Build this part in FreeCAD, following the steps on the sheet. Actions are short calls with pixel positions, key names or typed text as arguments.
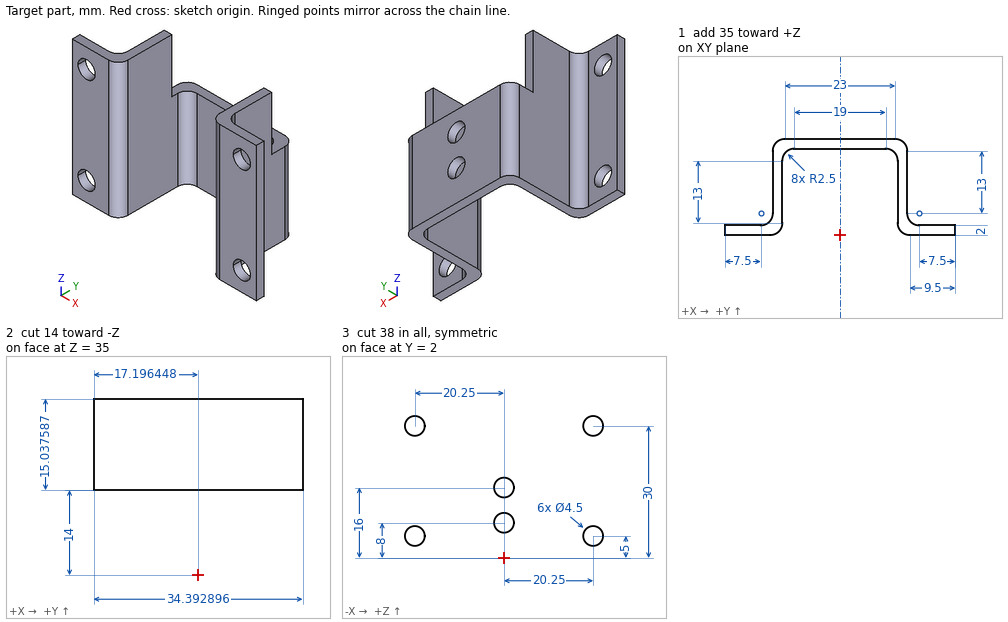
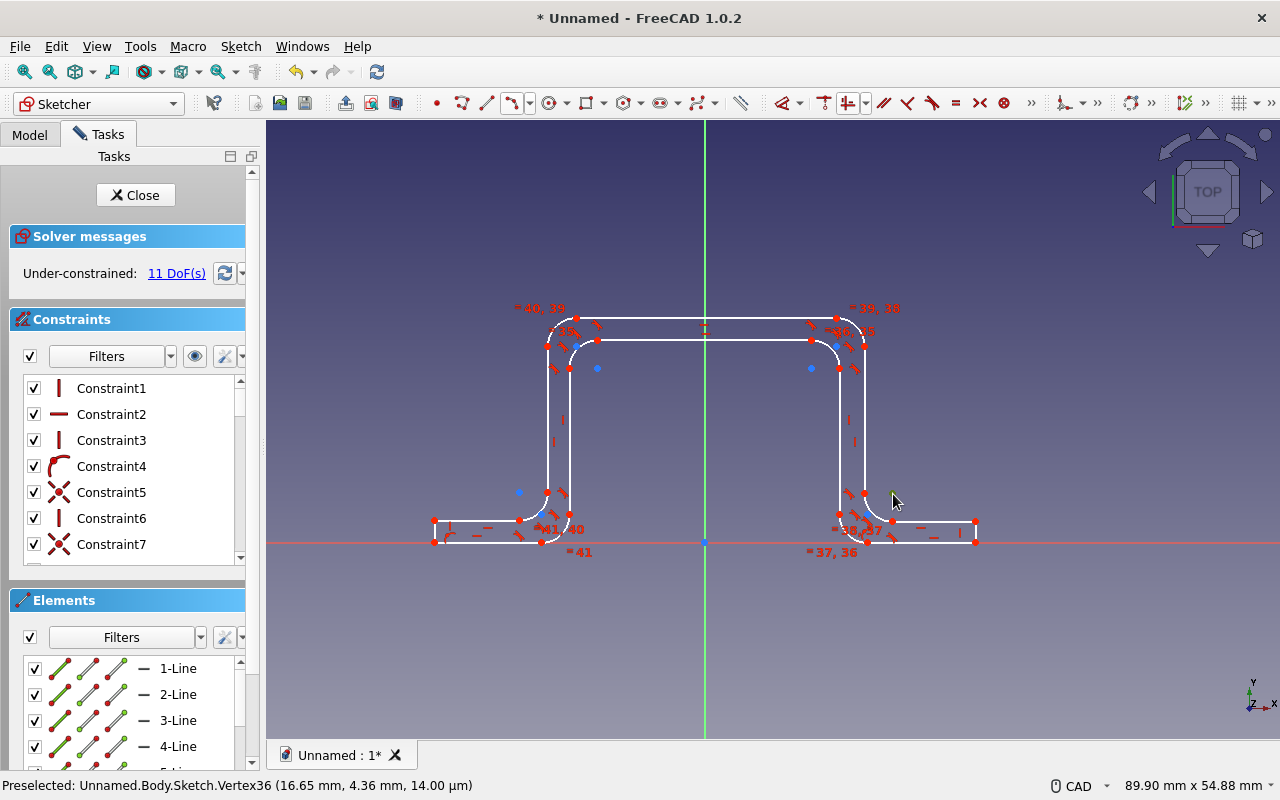
click(520, 492)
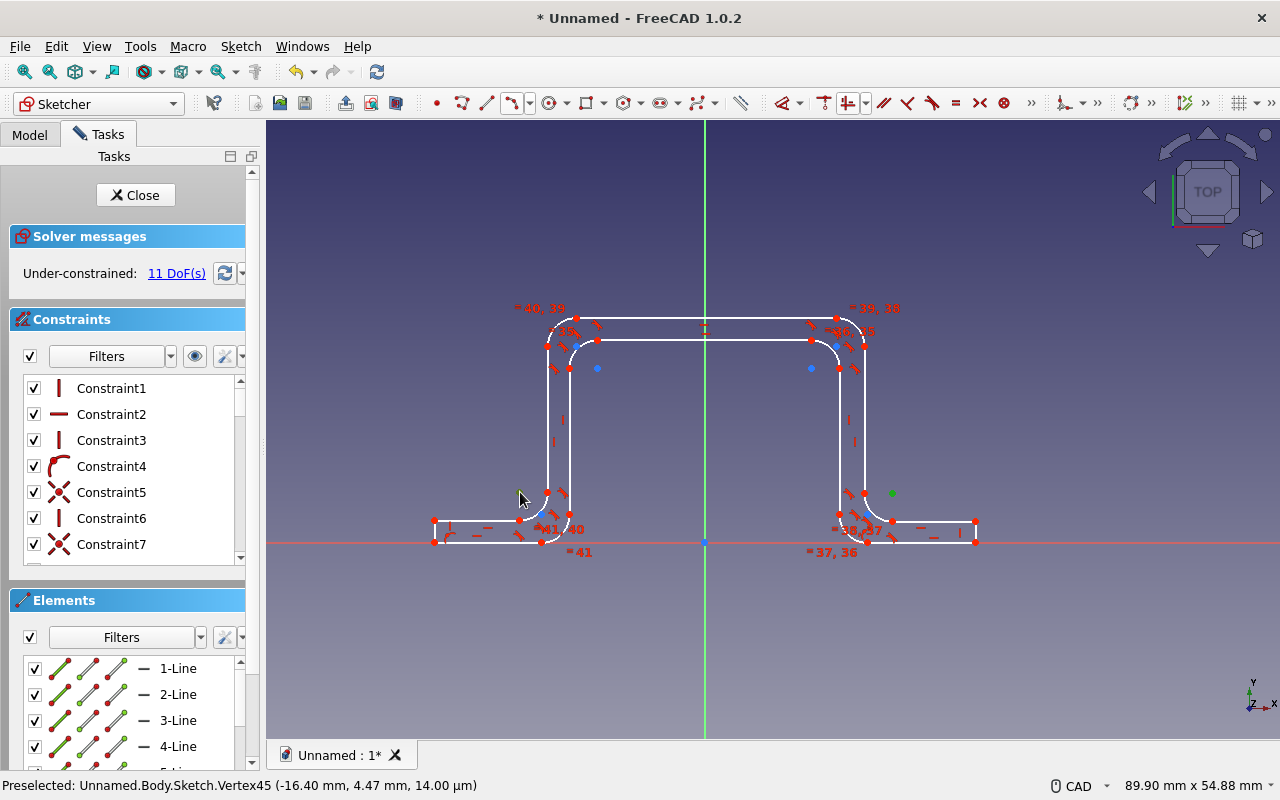
click(705, 671)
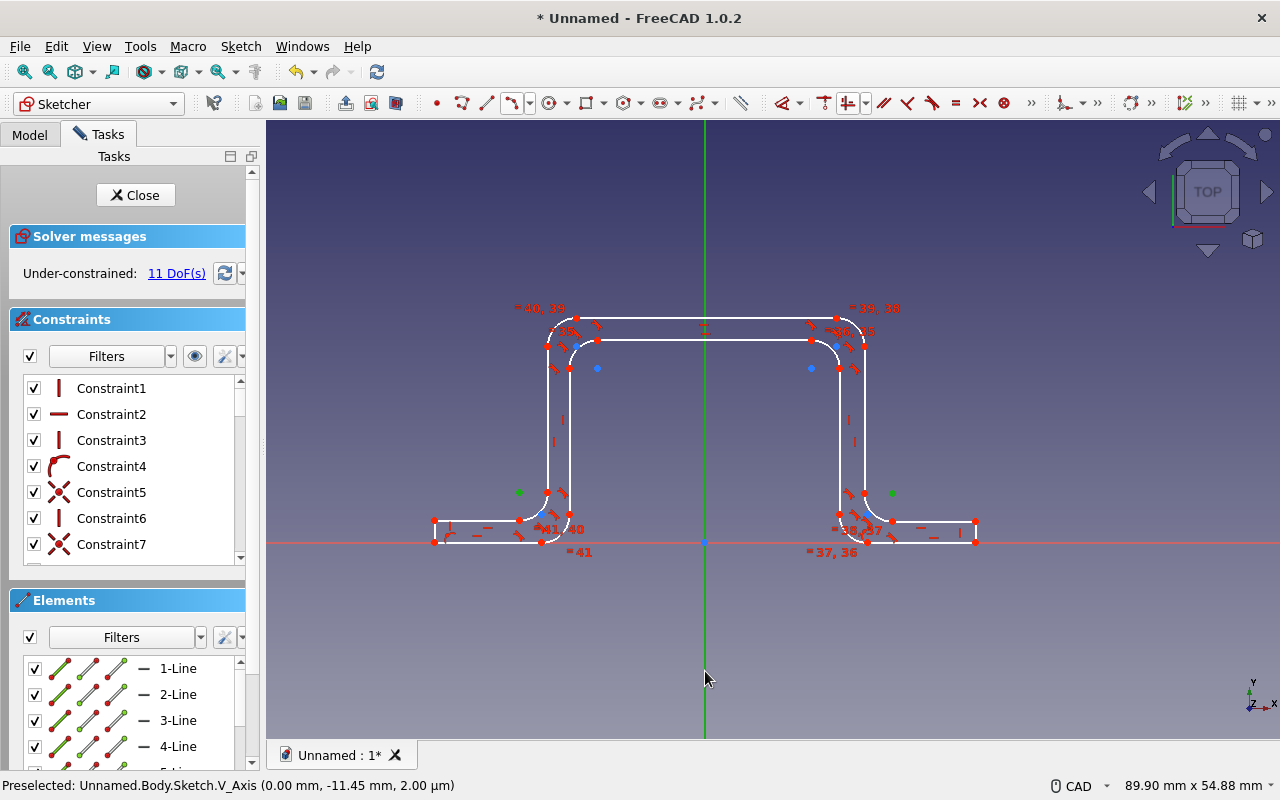
click(980, 104)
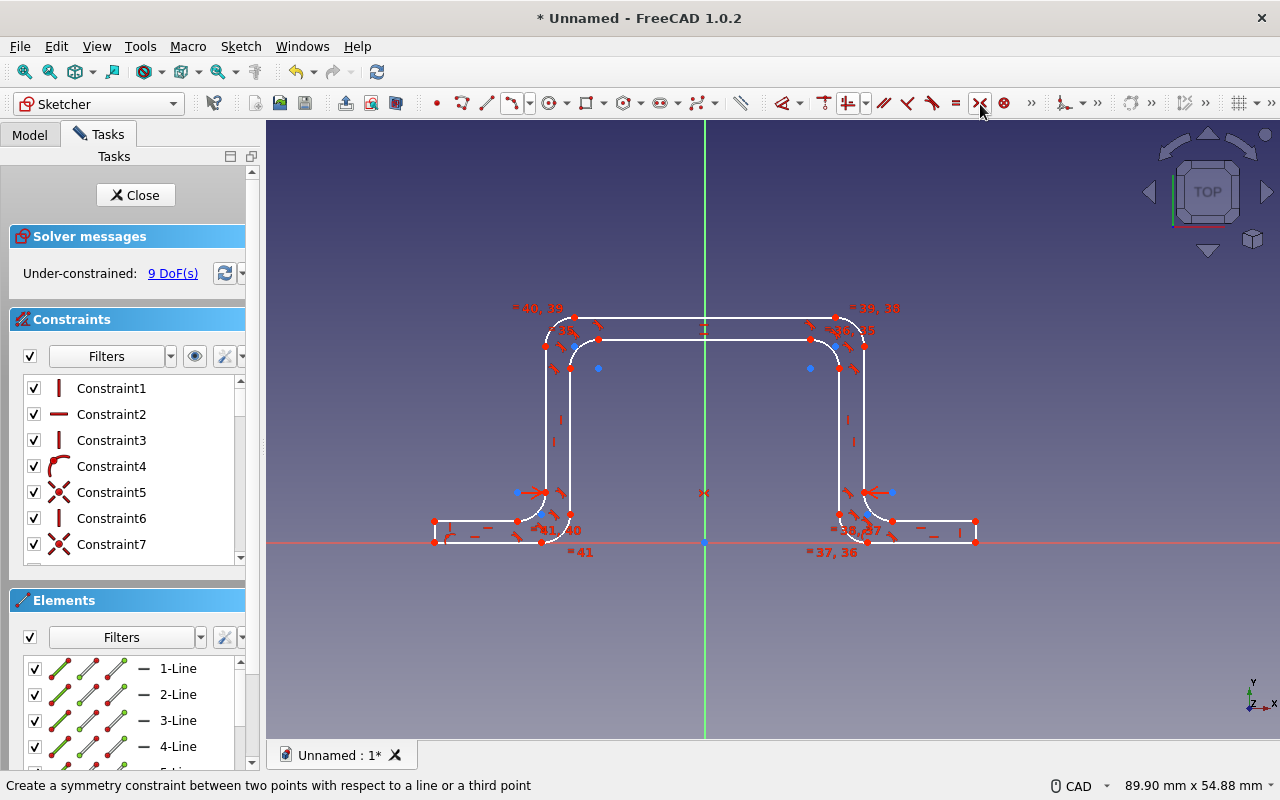
scroll(586, 343, up, 2)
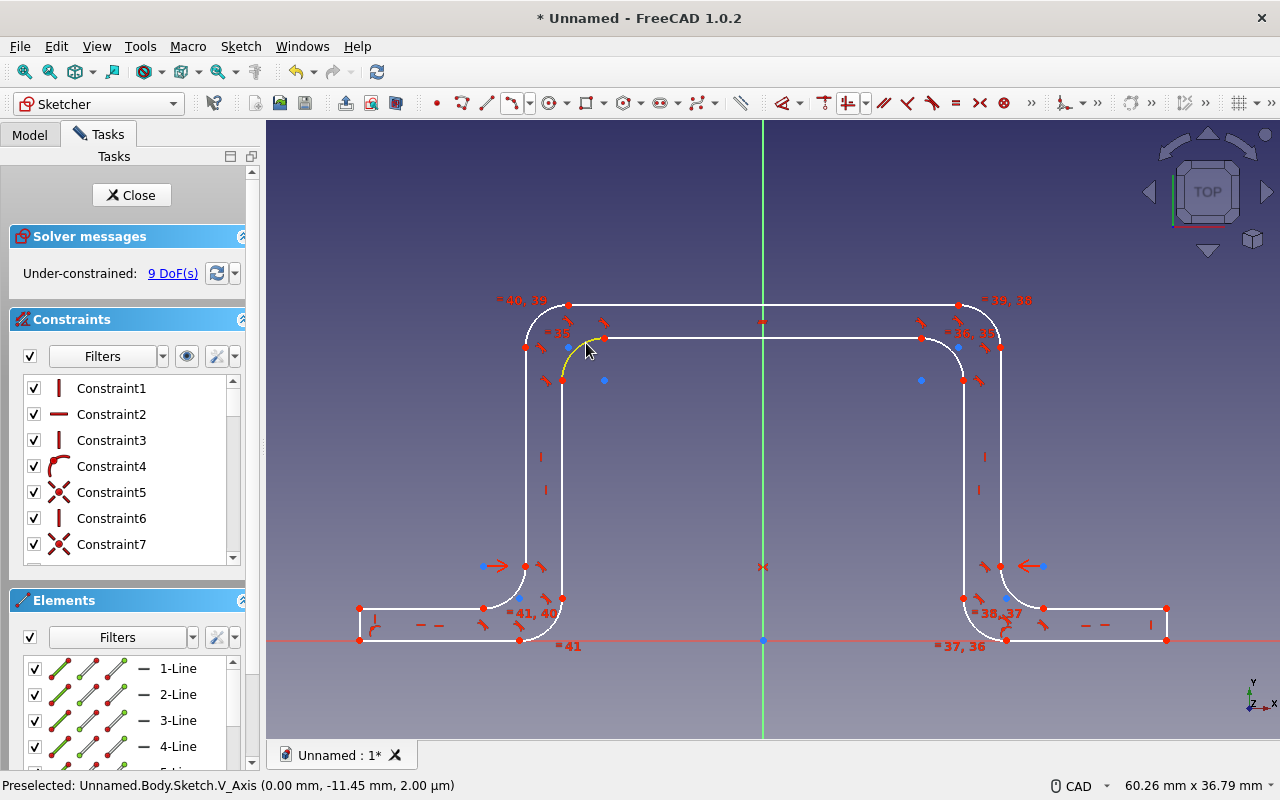
click(585, 343)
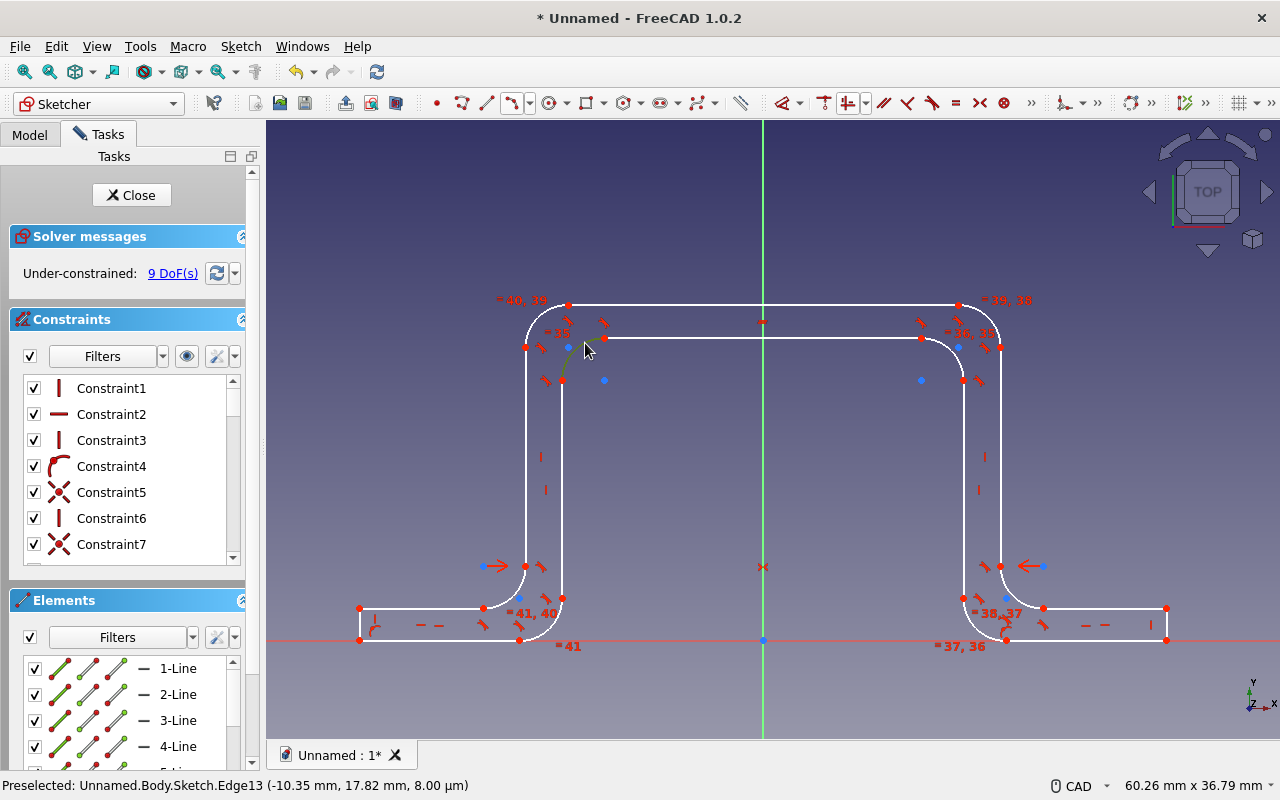
click(800, 104)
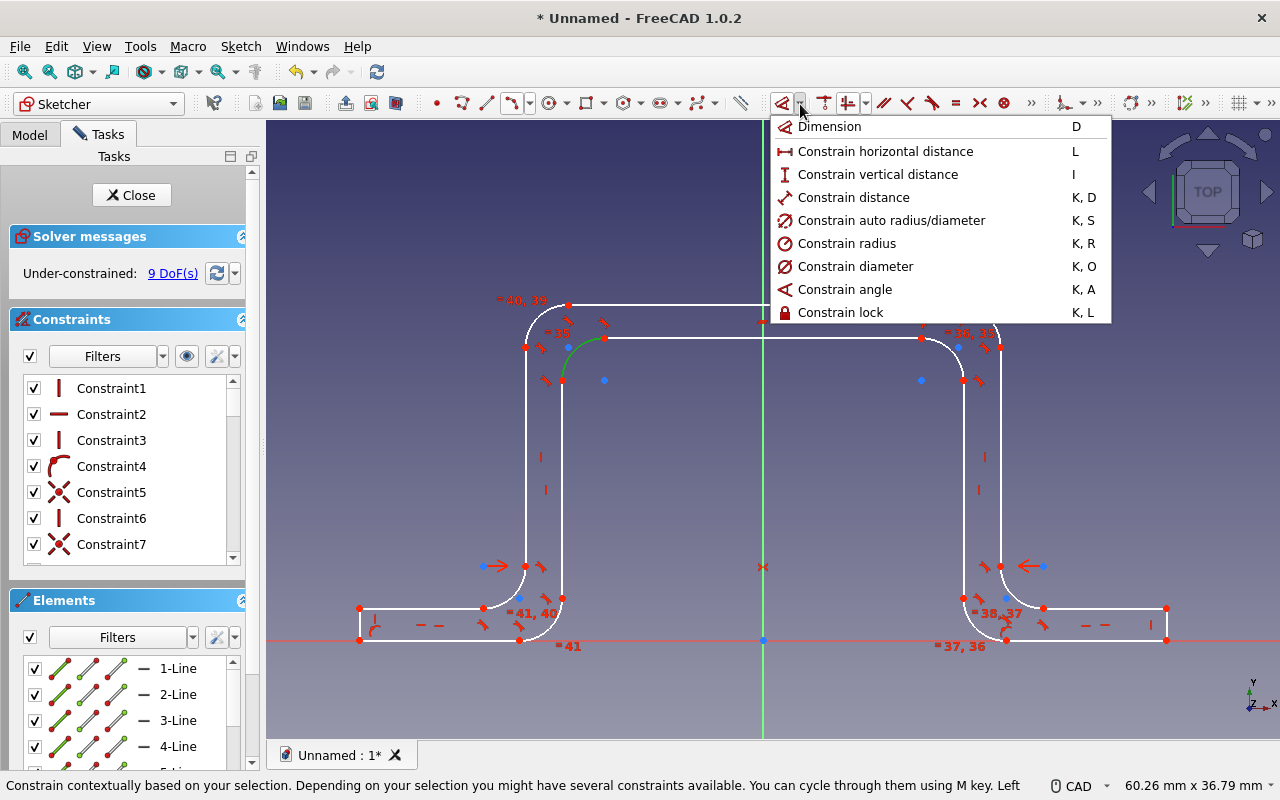
click(941, 244)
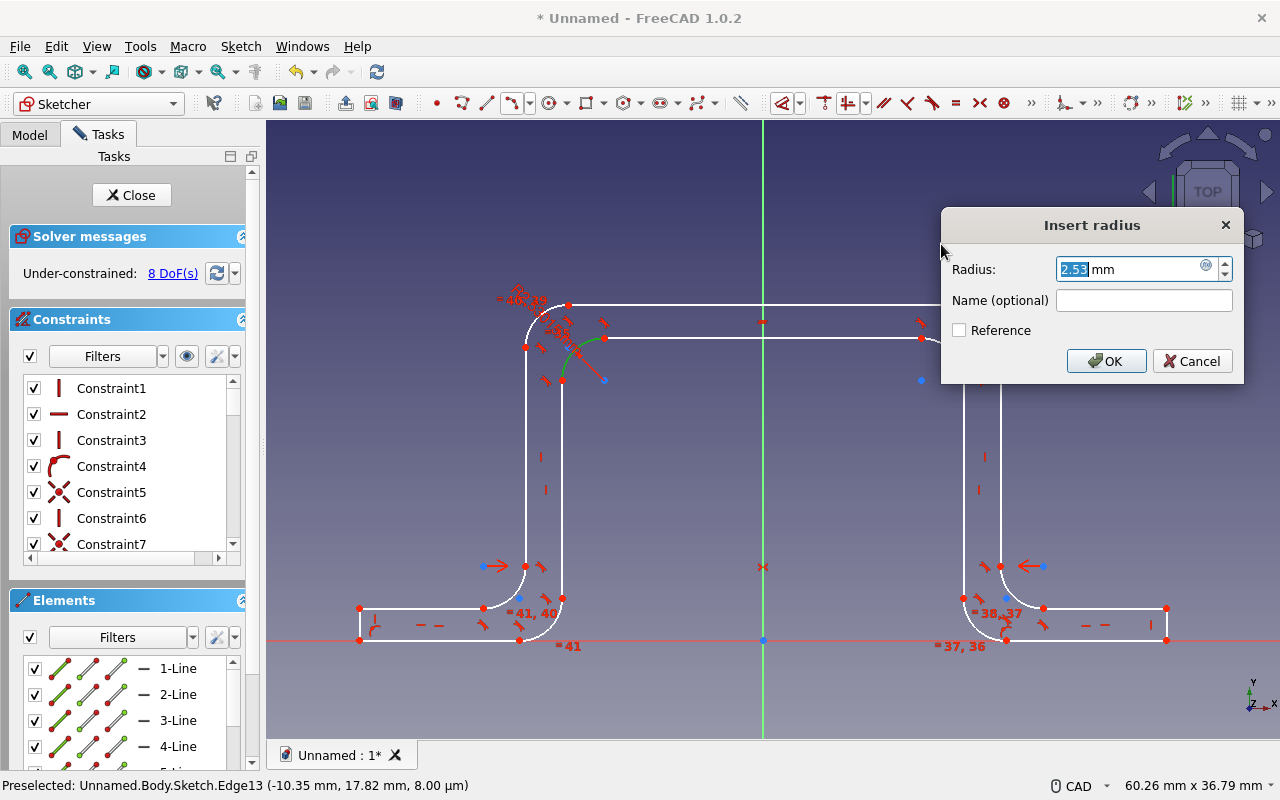
text(2.5)
key(Return)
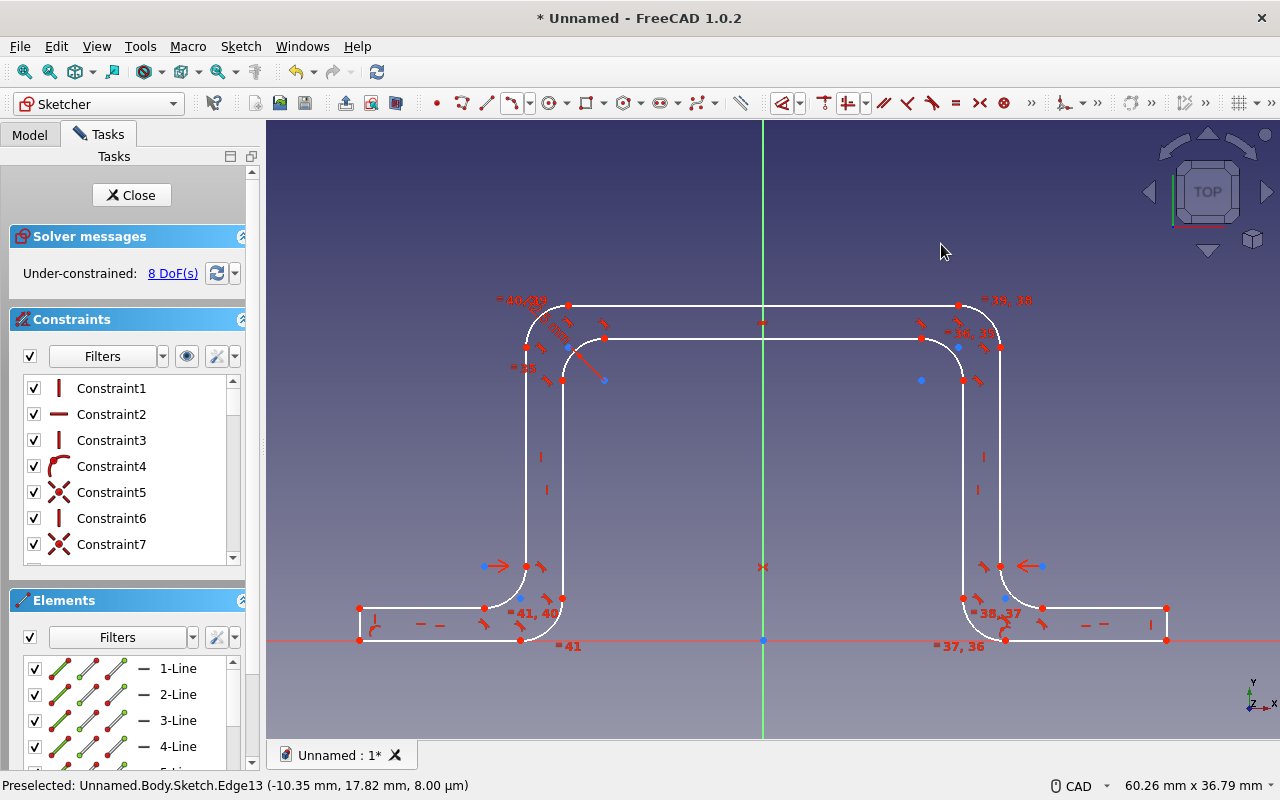
scroll(585, 342, down, 2)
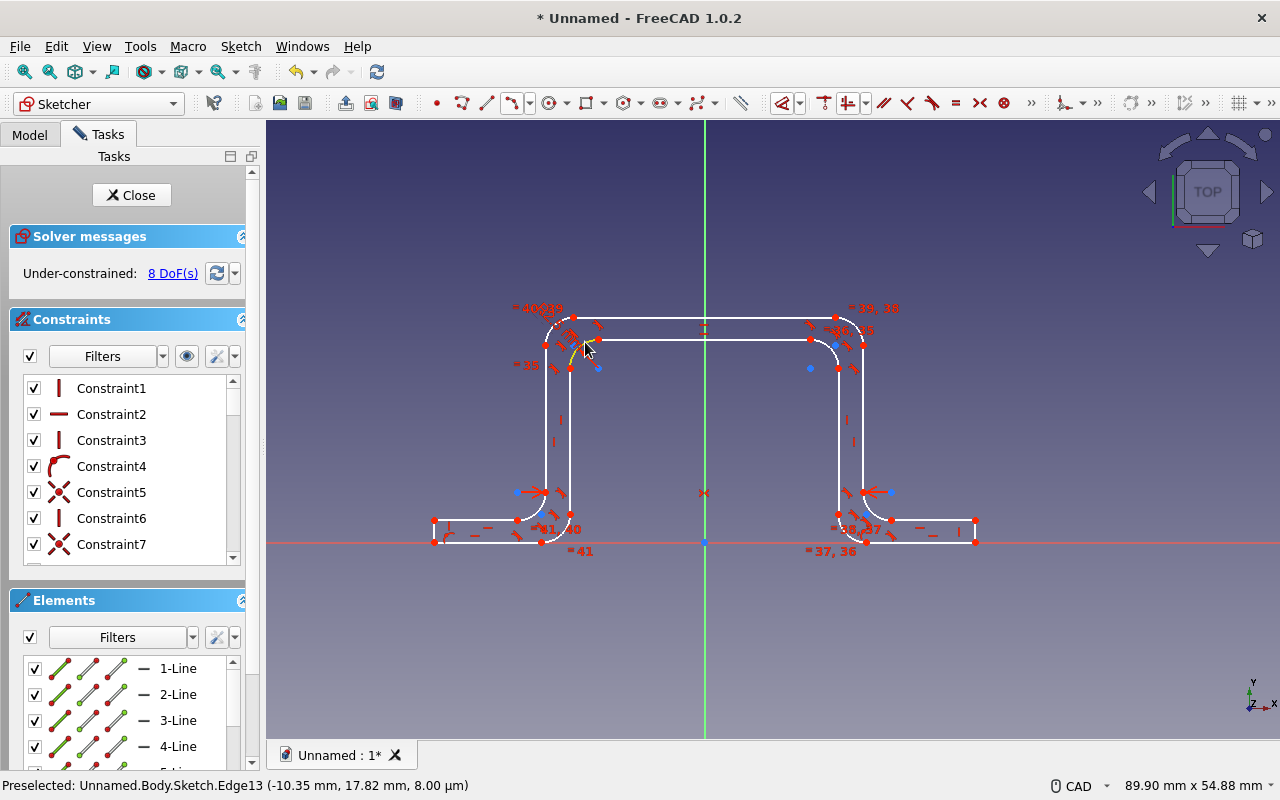
scroll(975, 536, up, 4)